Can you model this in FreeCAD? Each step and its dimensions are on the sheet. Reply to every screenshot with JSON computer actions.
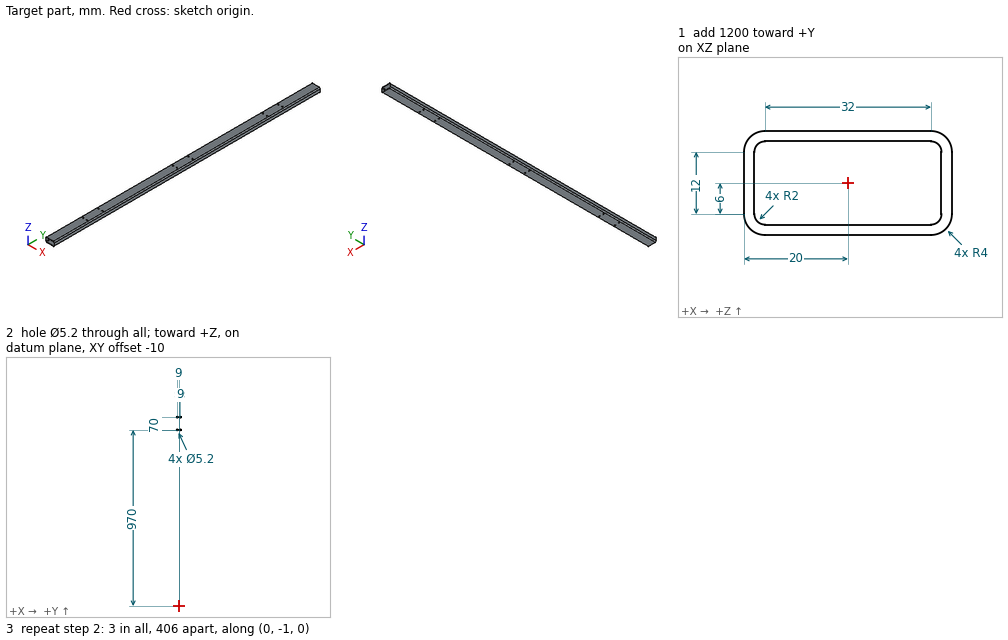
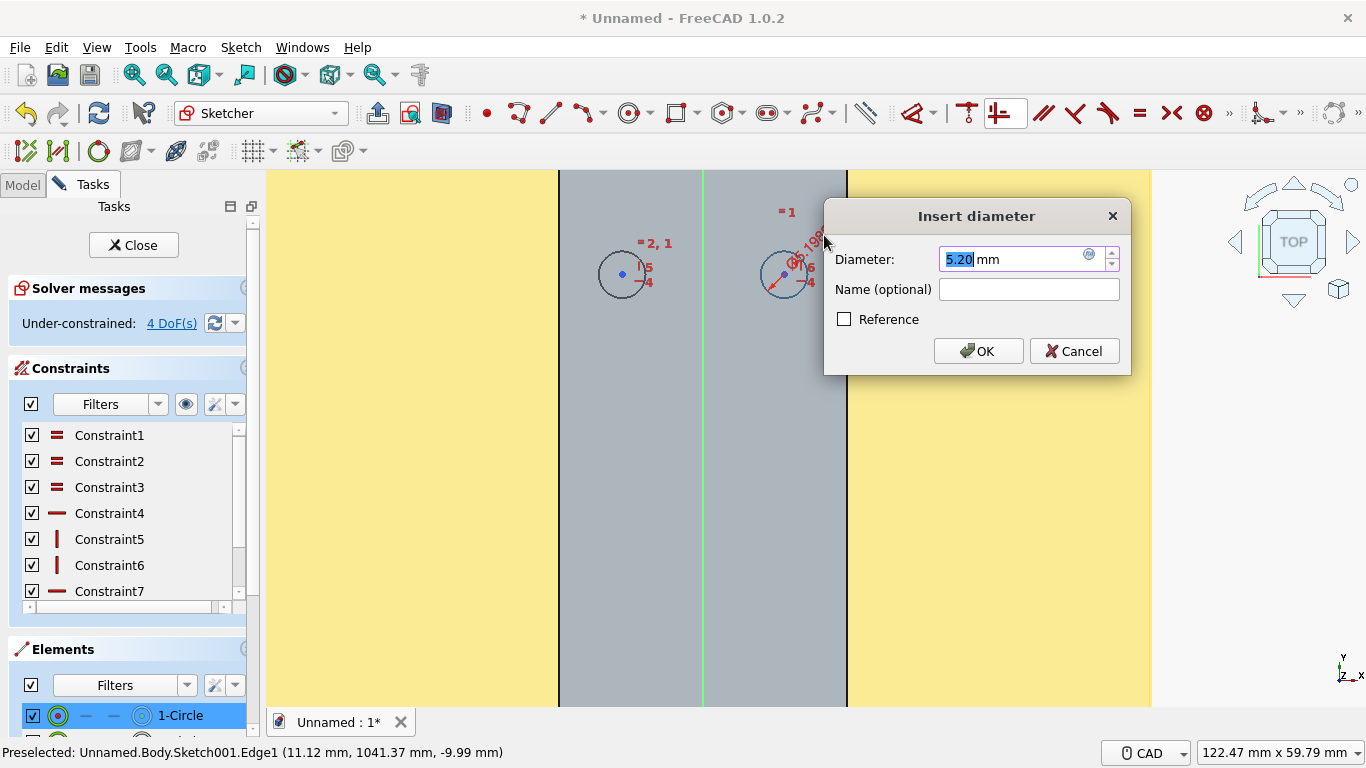
{"action": "type", "text": "5.2"}
{"action": "key", "text": "Return"}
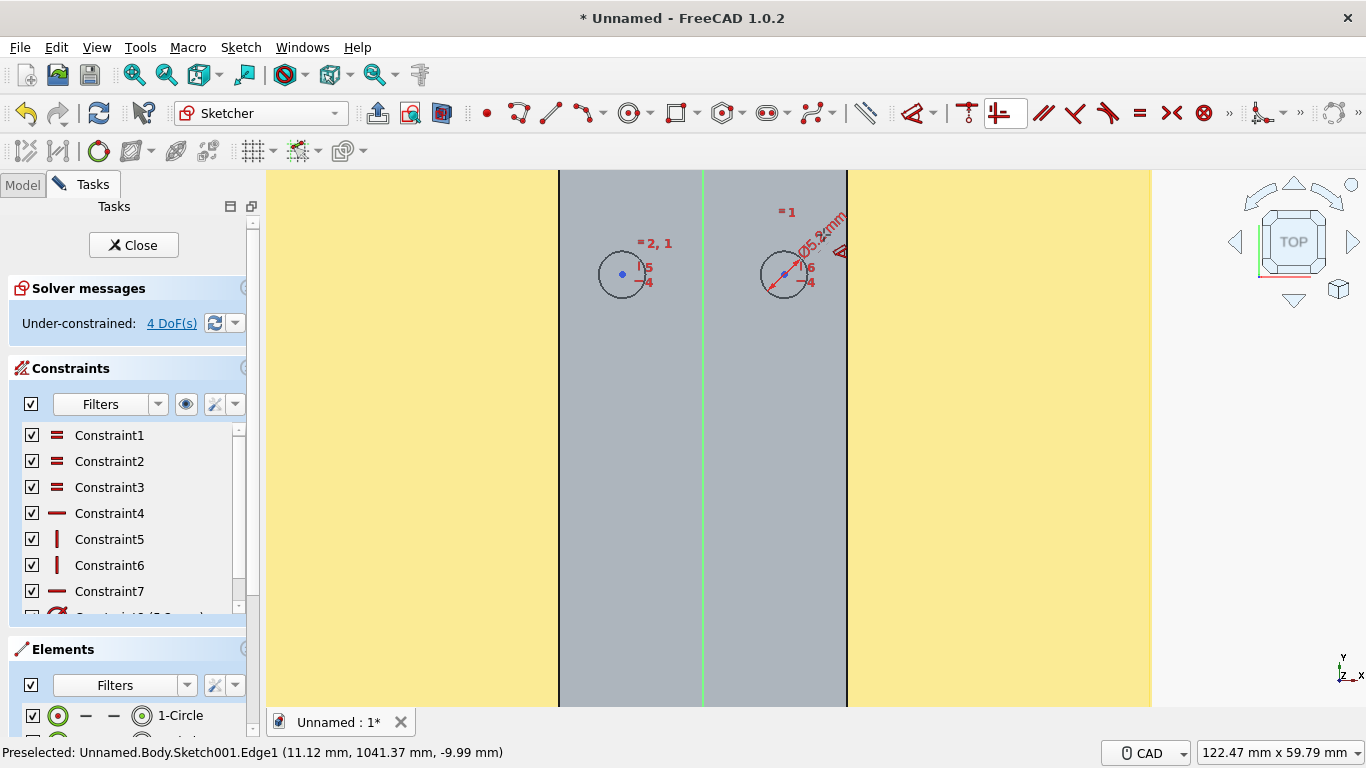
{"action": "left_click", "coordinate": [784, 275]}
{"action": "left_click", "coordinate": [744, 241]}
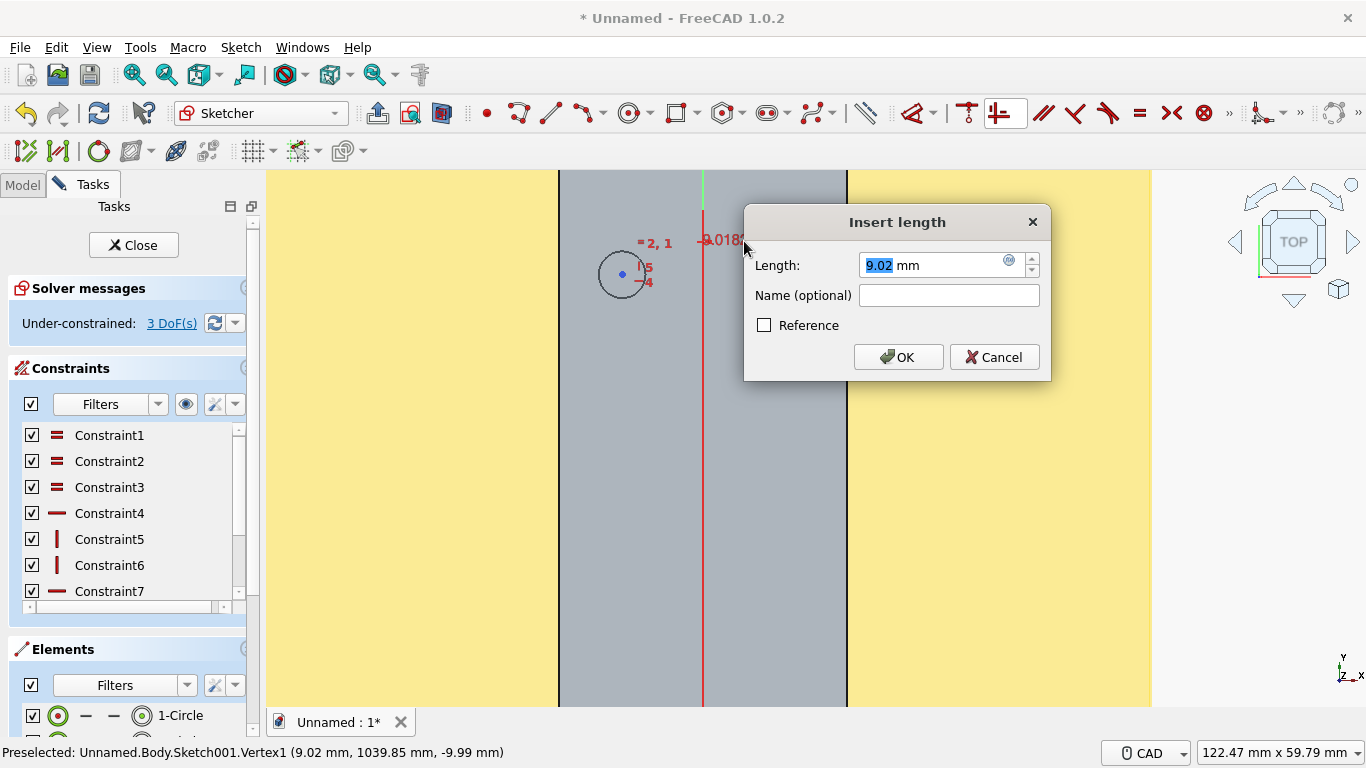
{"action": "type", "text": "9"}
{"action": "key", "text": "Return"}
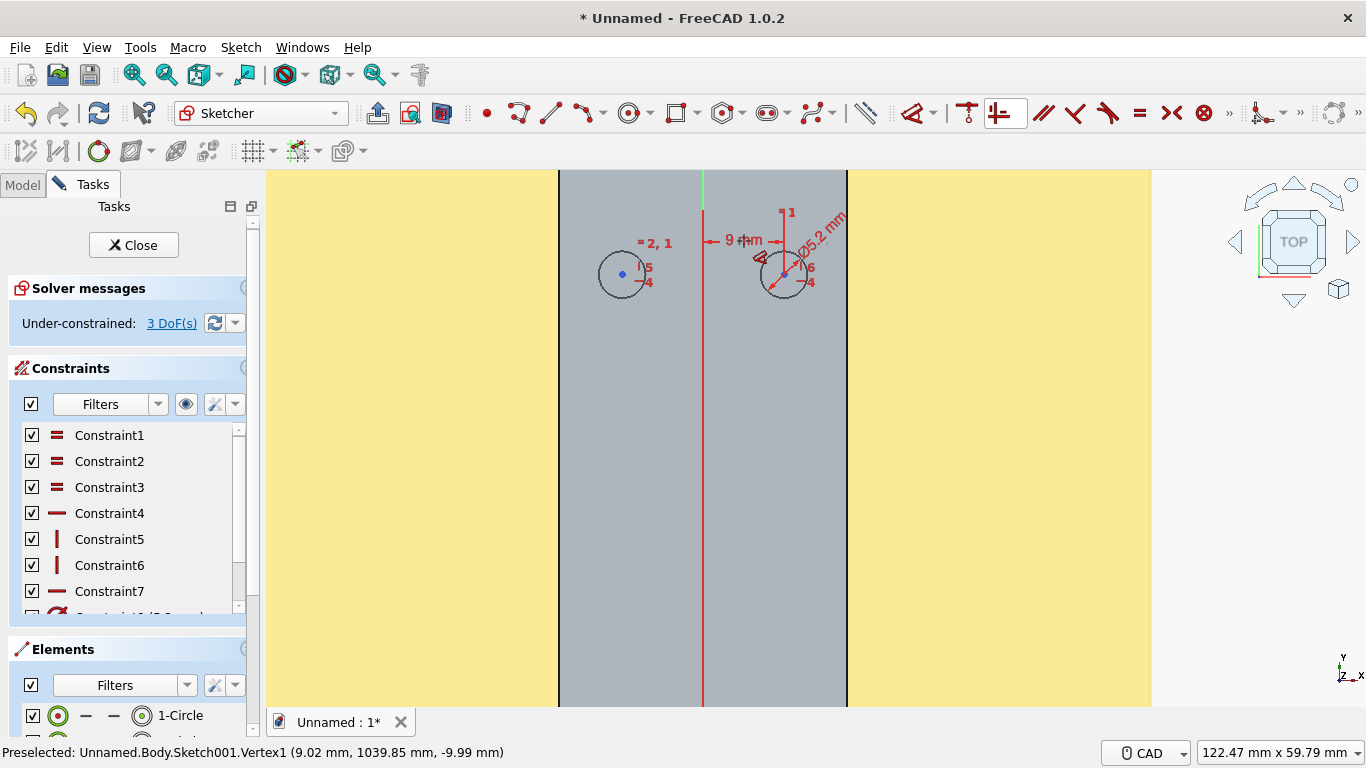
{"action": "left_click", "coordinate": [622, 275]}
{"action": "left_click", "coordinate": [663, 241]}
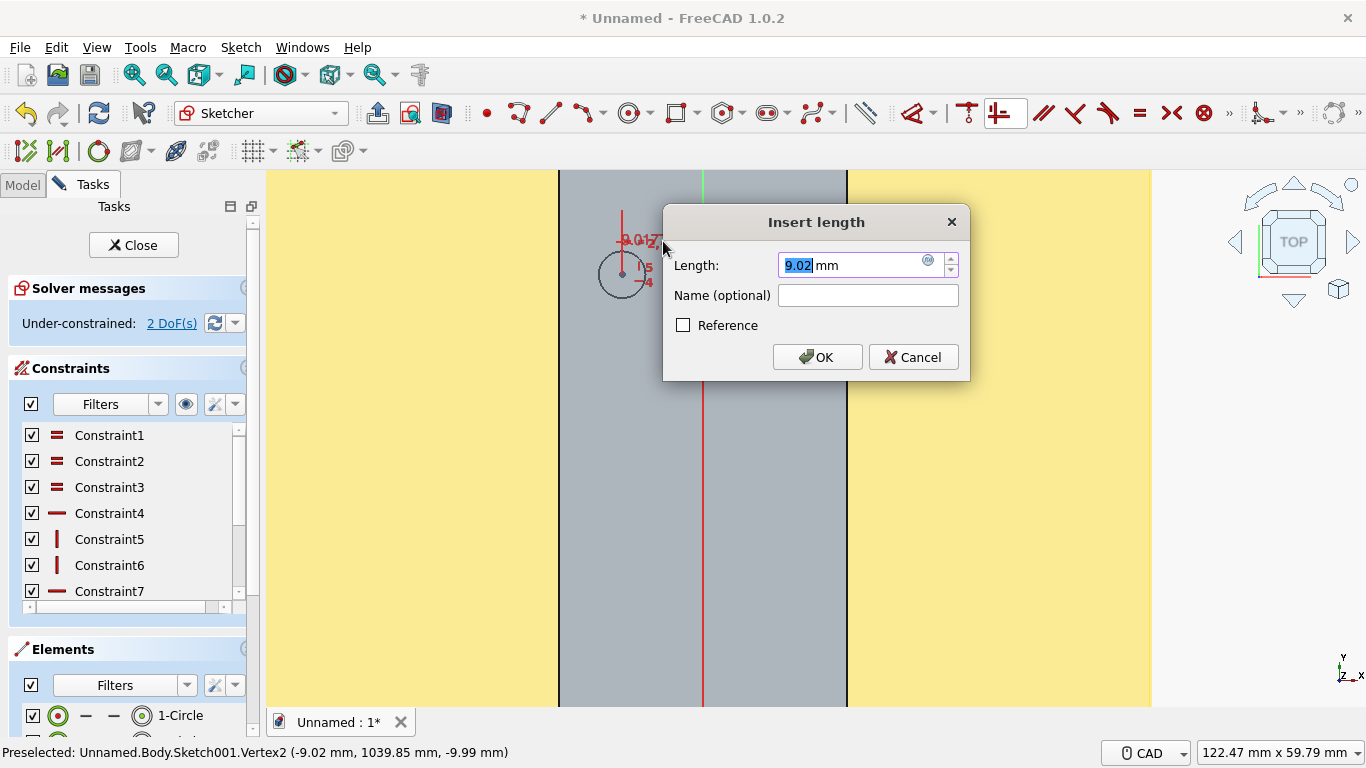
{"action": "type", "text": "9"}
{"action": "key", "text": "Return"}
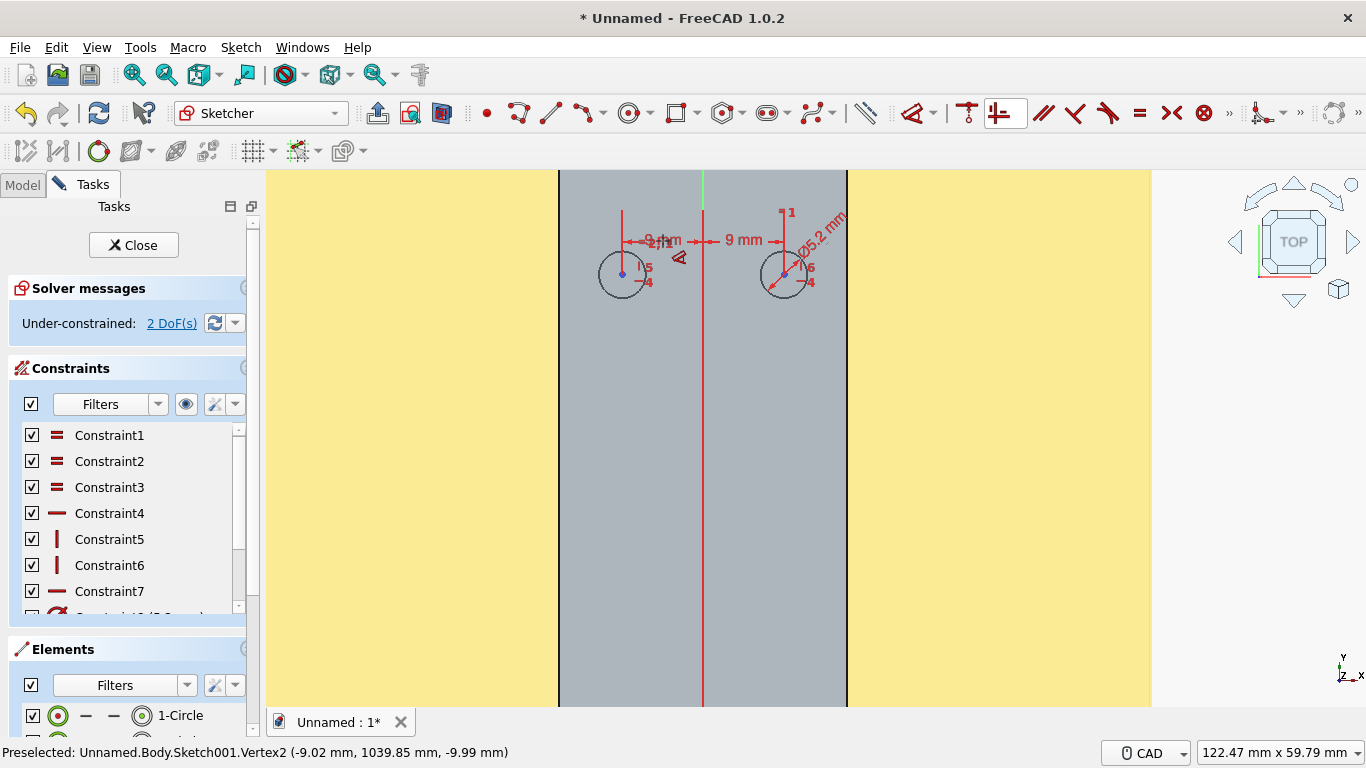
{"action": "scroll", "coordinate": [801, 257], "scroll_direction": "down", "scroll_amount": 3}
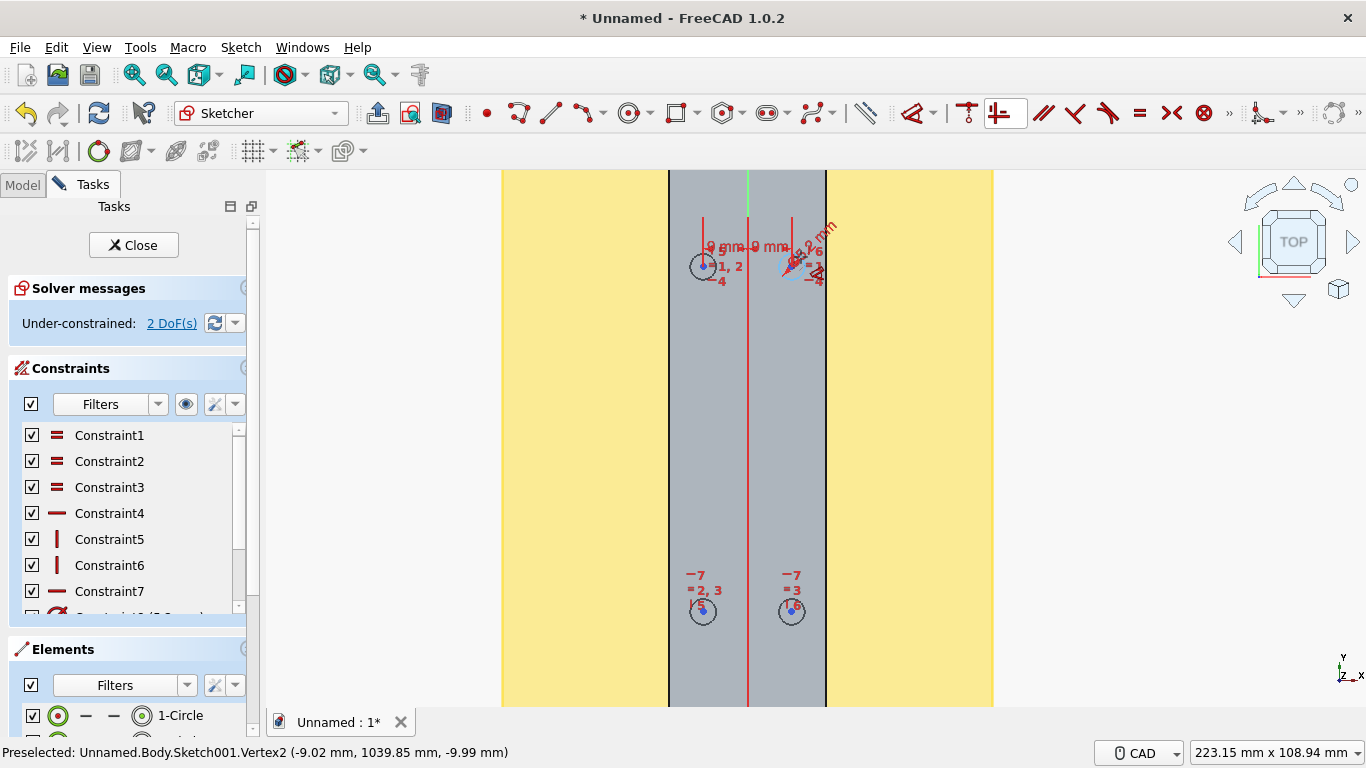
{"action": "left_click", "coordinate": [703, 612]}
{"action": "left_click", "coordinate": [669, 645]}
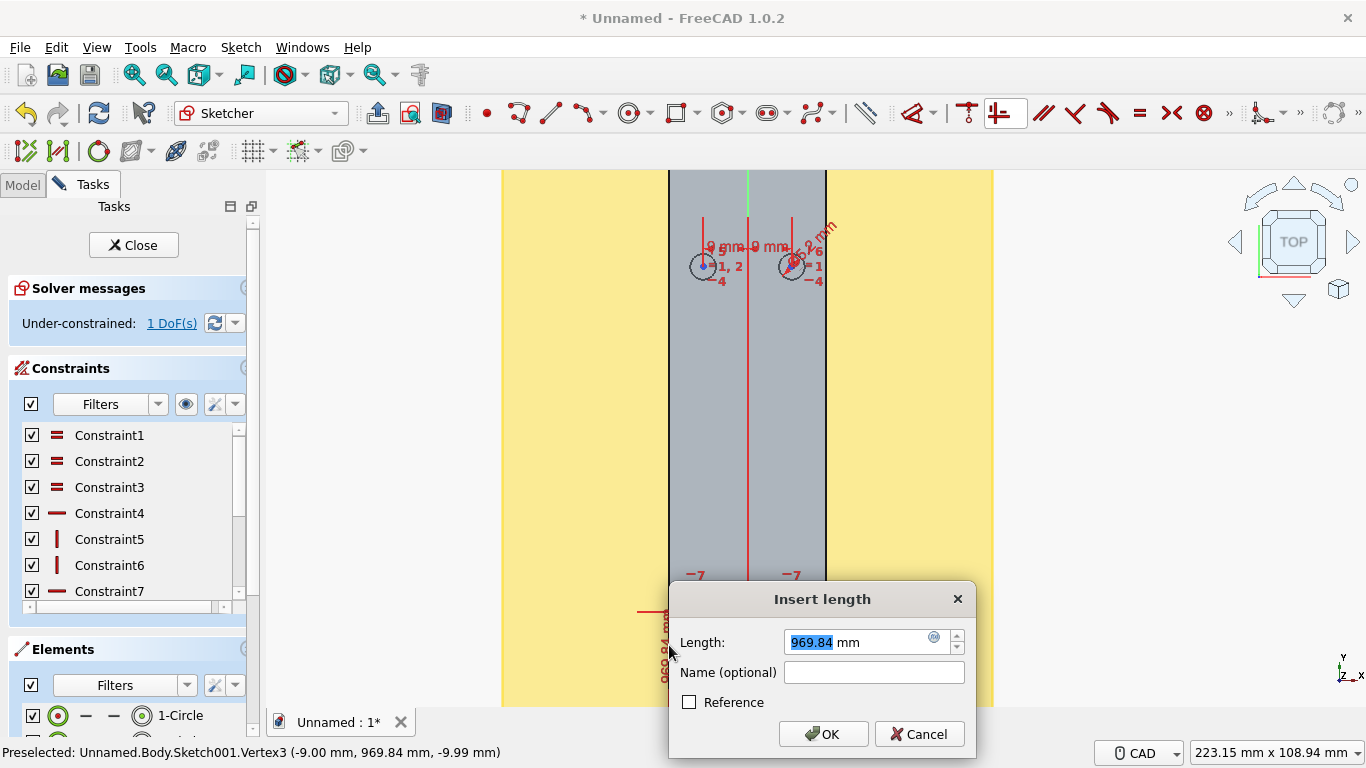
{"action": "type", "text": "970"}
{"action": "key", "text": "Return"}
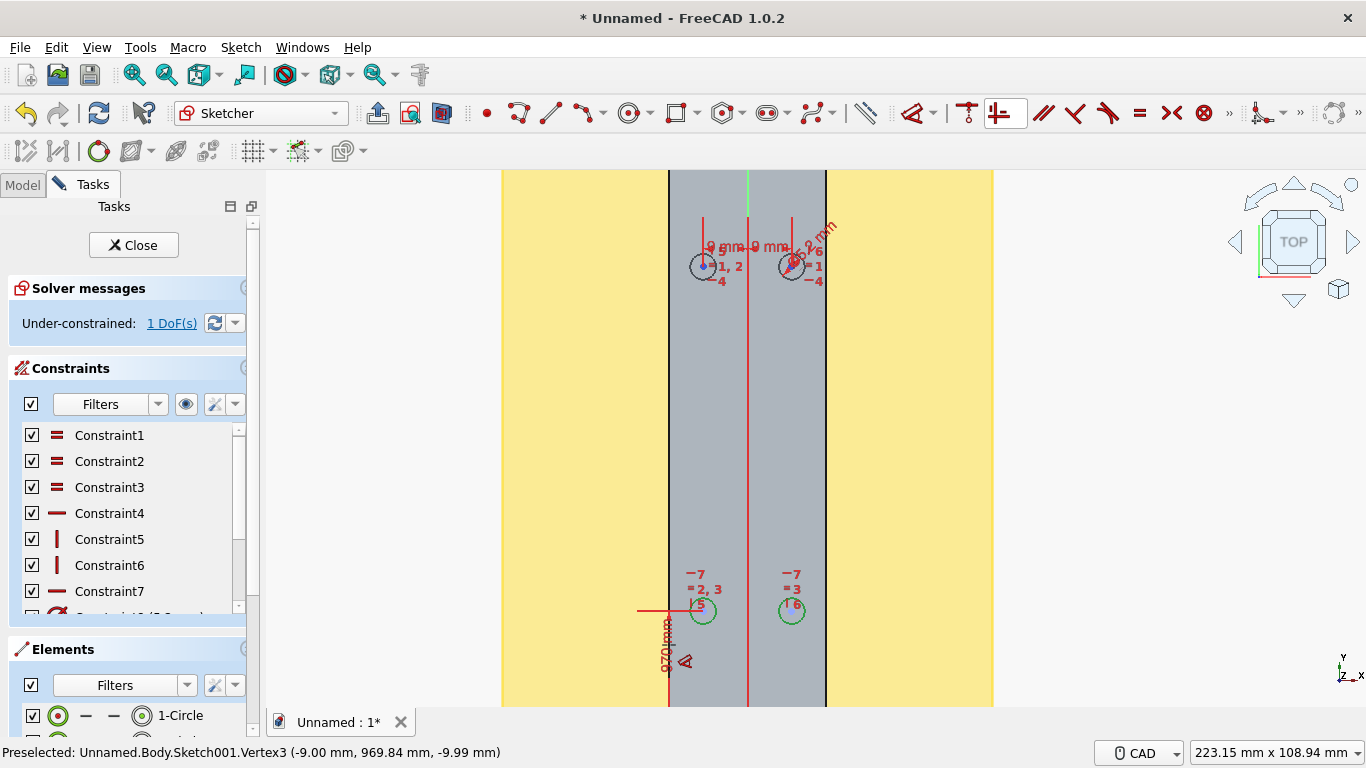
{"action": "left_click", "coordinate": [703, 267]}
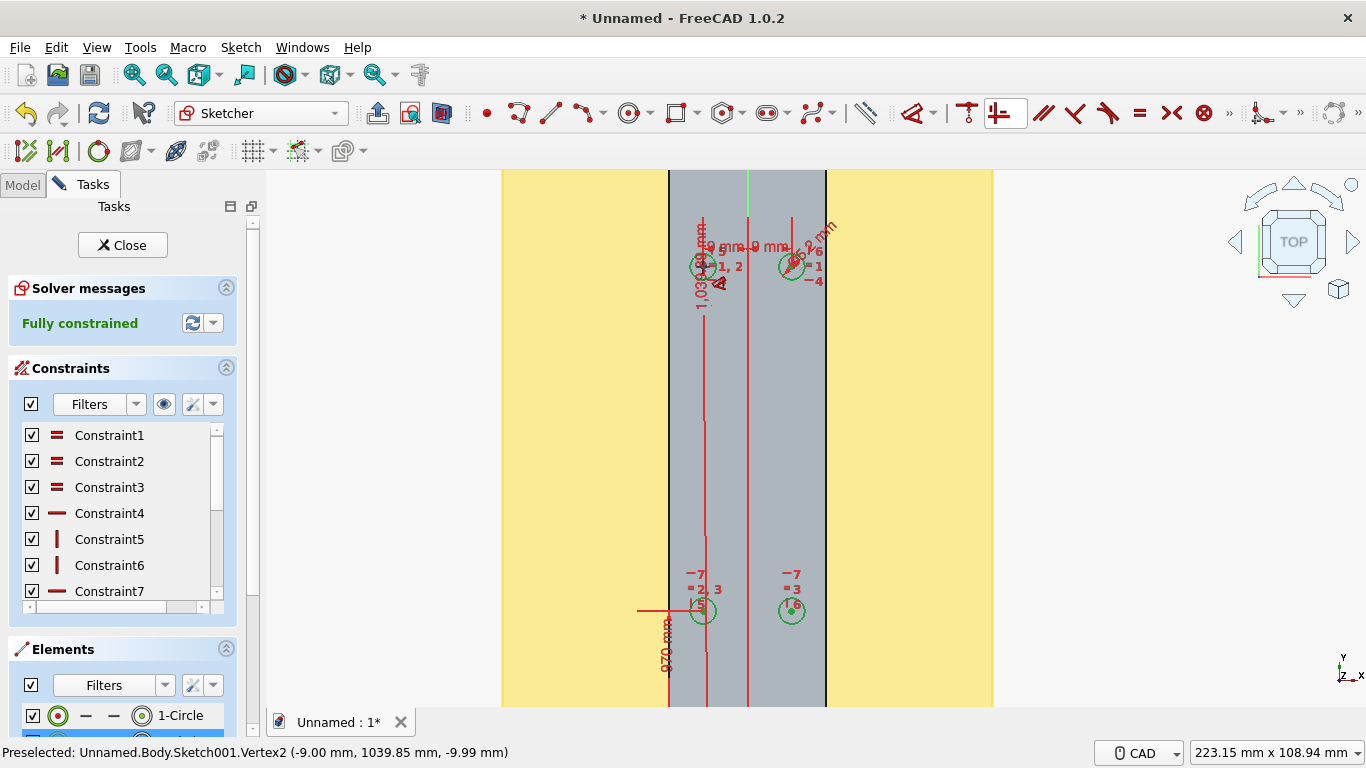
{"action": "left_click", "coordinate": [703, 611]}
{"action": "left_click", "coordinate": [669, 439]}